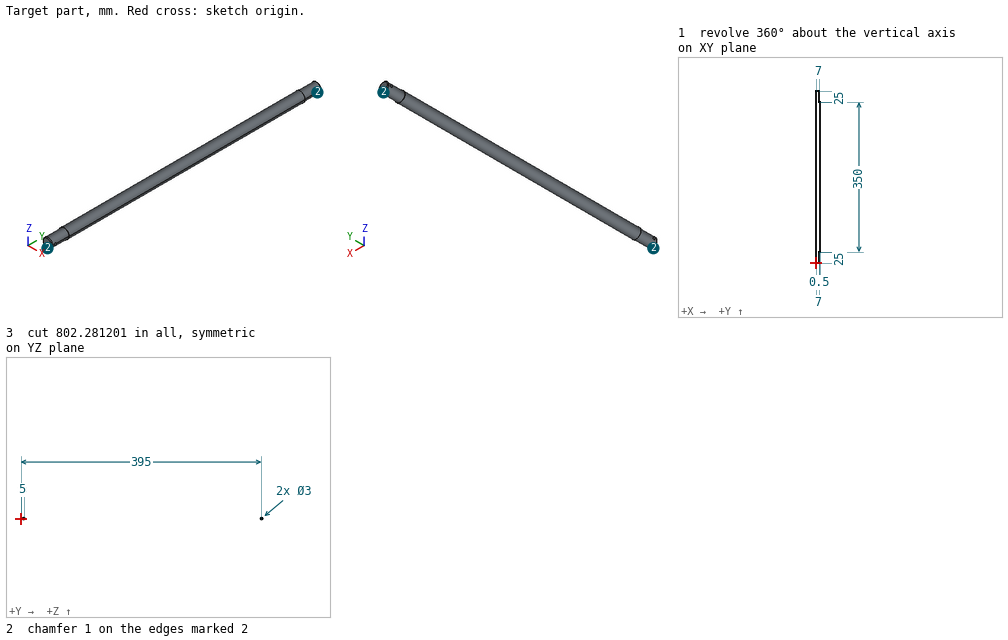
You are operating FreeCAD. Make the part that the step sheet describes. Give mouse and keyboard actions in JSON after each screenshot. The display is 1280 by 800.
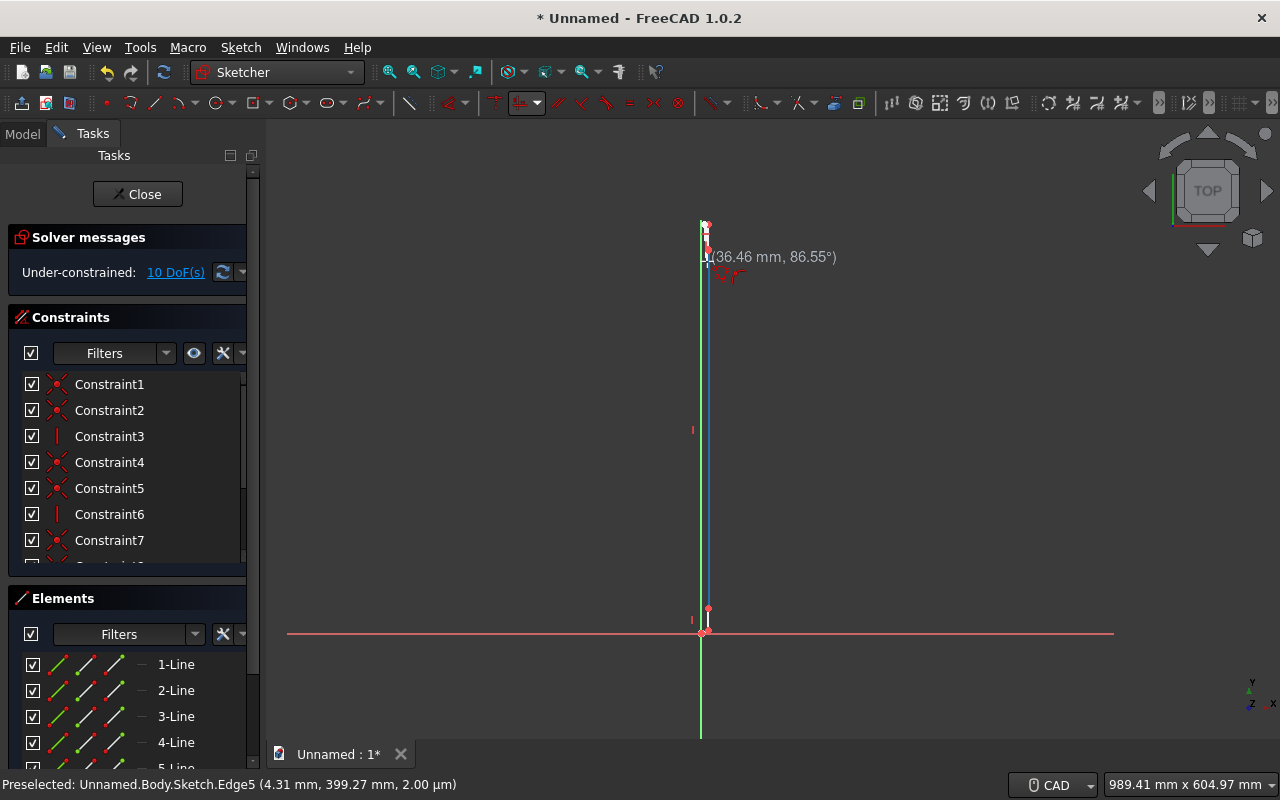
{"action": "scroll", "coordinate": [701, 634], "scroll_direction": "up", "scroll_amount": 8}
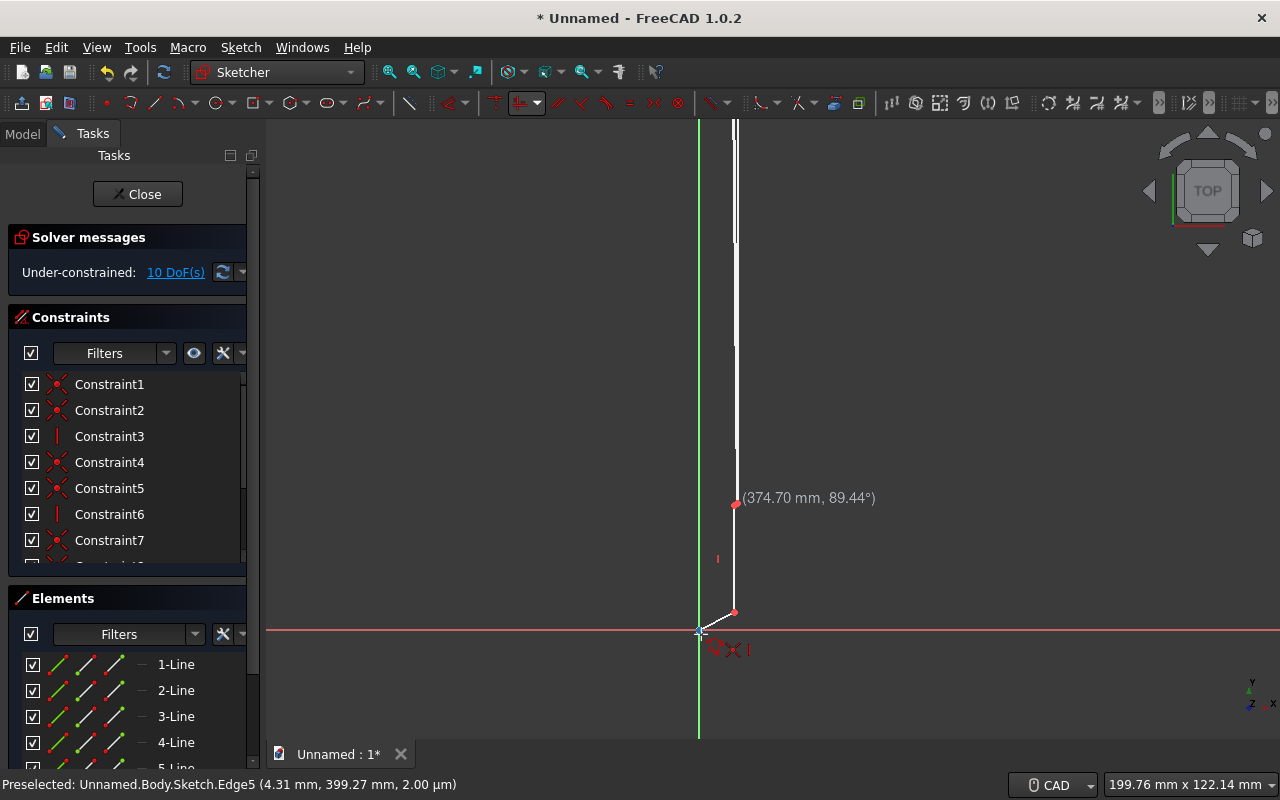
{"action": "left_click", "coordinate": [699, 630]}
{"action": "key", "text": "Escape"}
{"action": "key", "text": "Escape"}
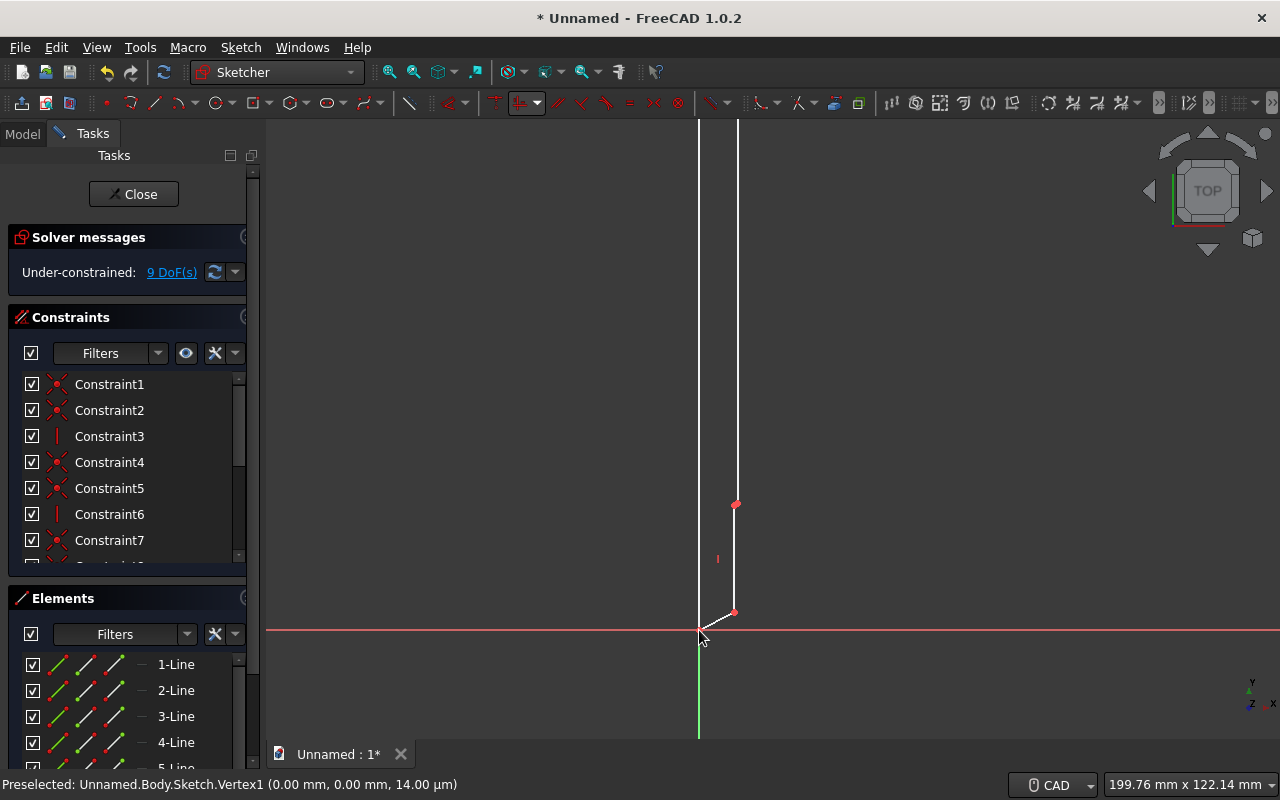
{"action": "left_click", "coordinate": [724, 618]}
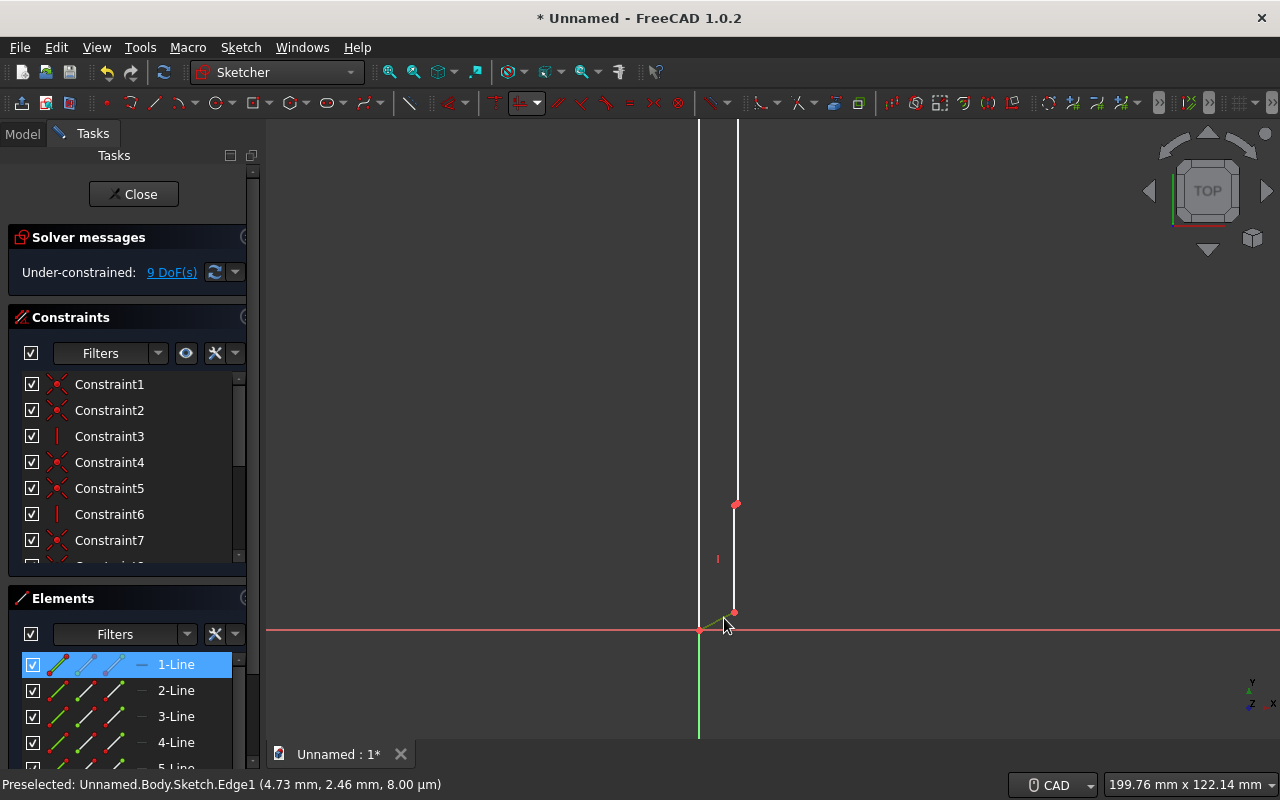
{"action": "left_click", "coordinate": [540, 104]}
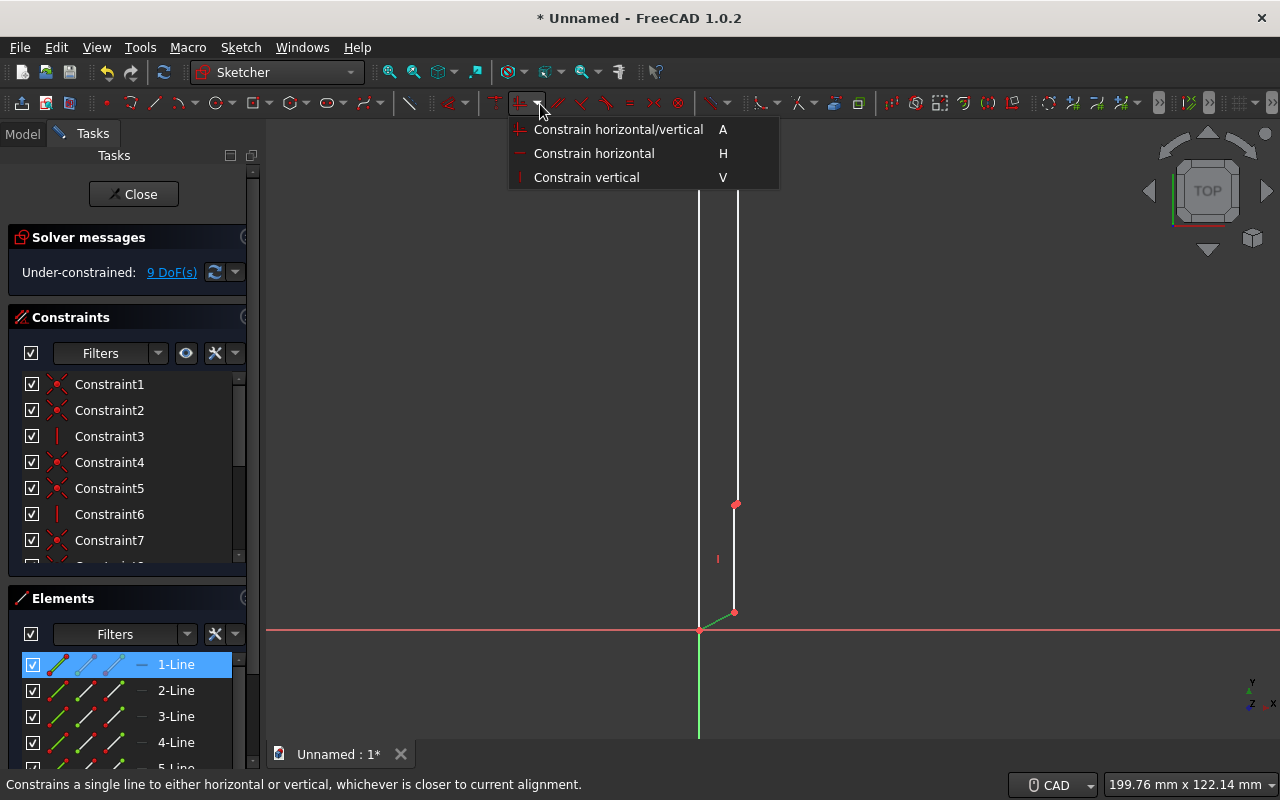
{"action": "left_click", "coordinate": [644, 153]}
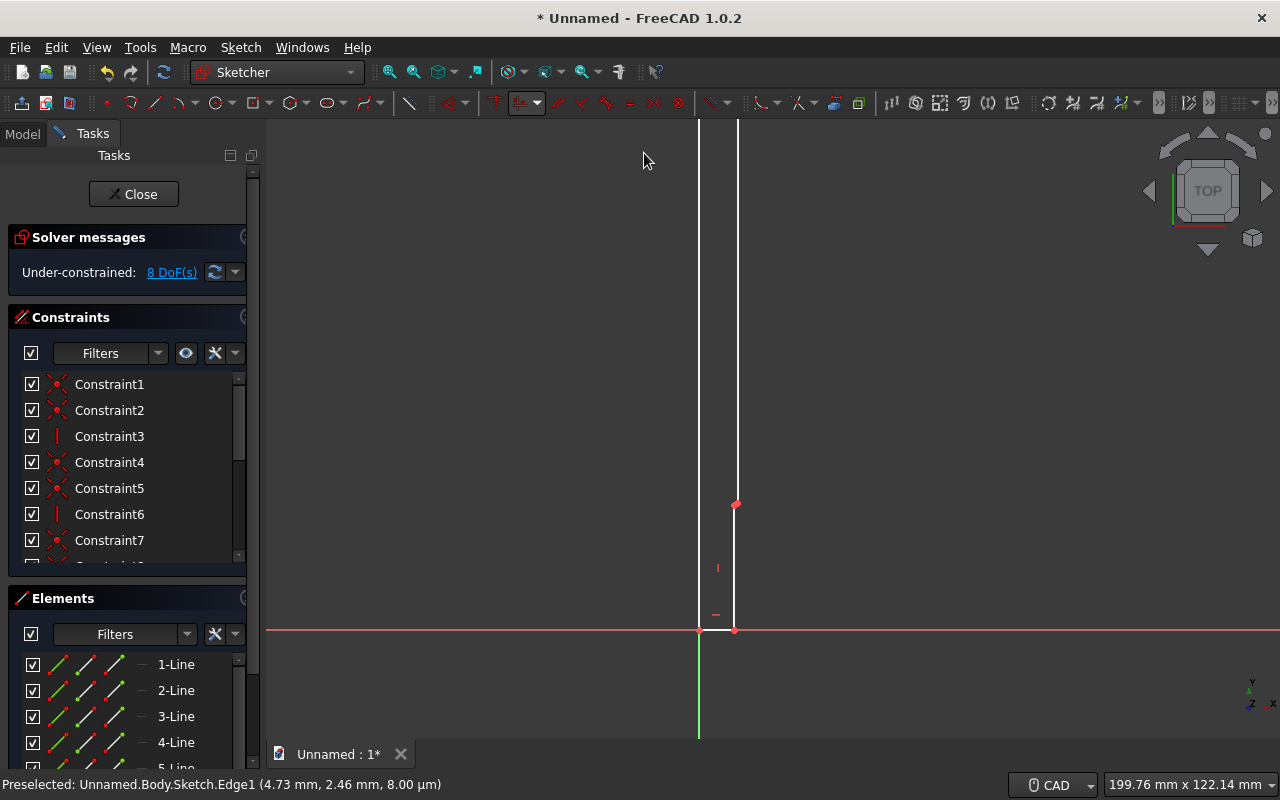
{"action": "scroll", "coordinate": [736, 504], "scroll_direction": "up", "scroll_amount": 6}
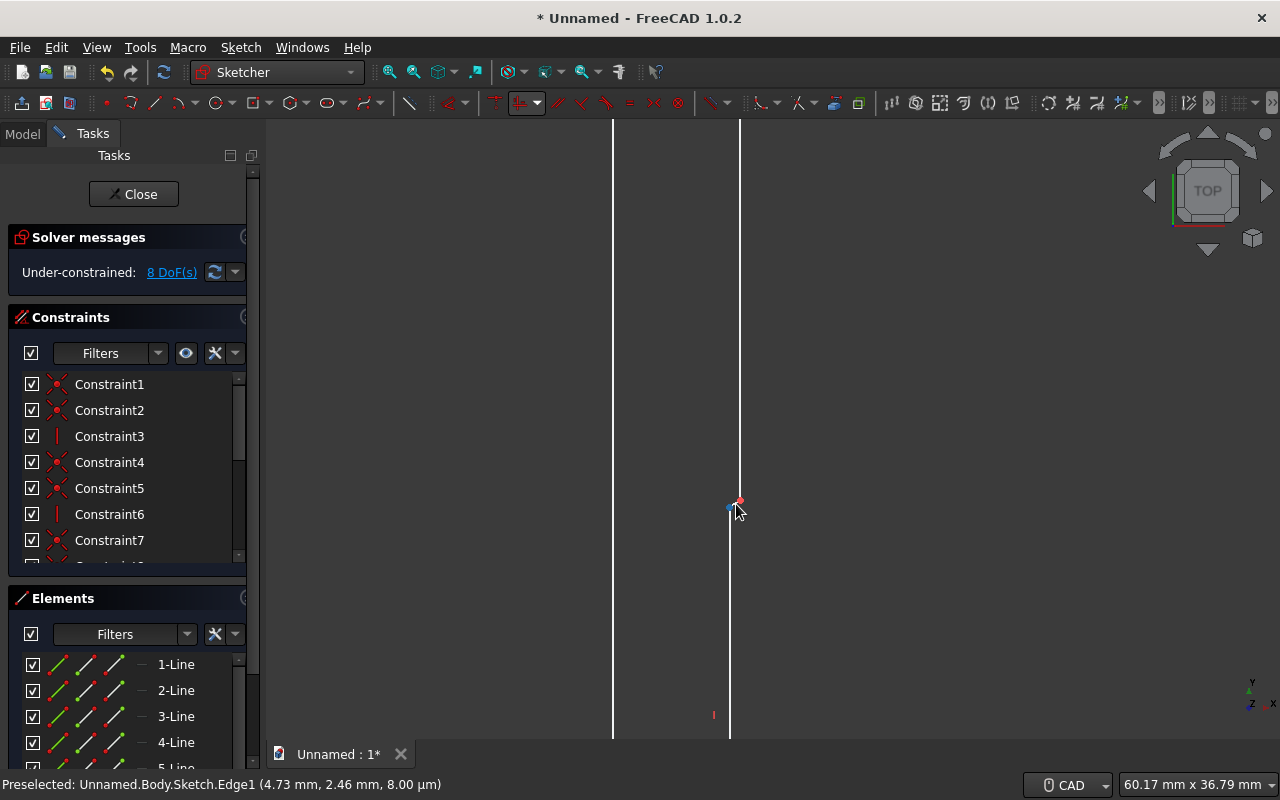
{"action": "left_click", "coordinate": [735, 504]}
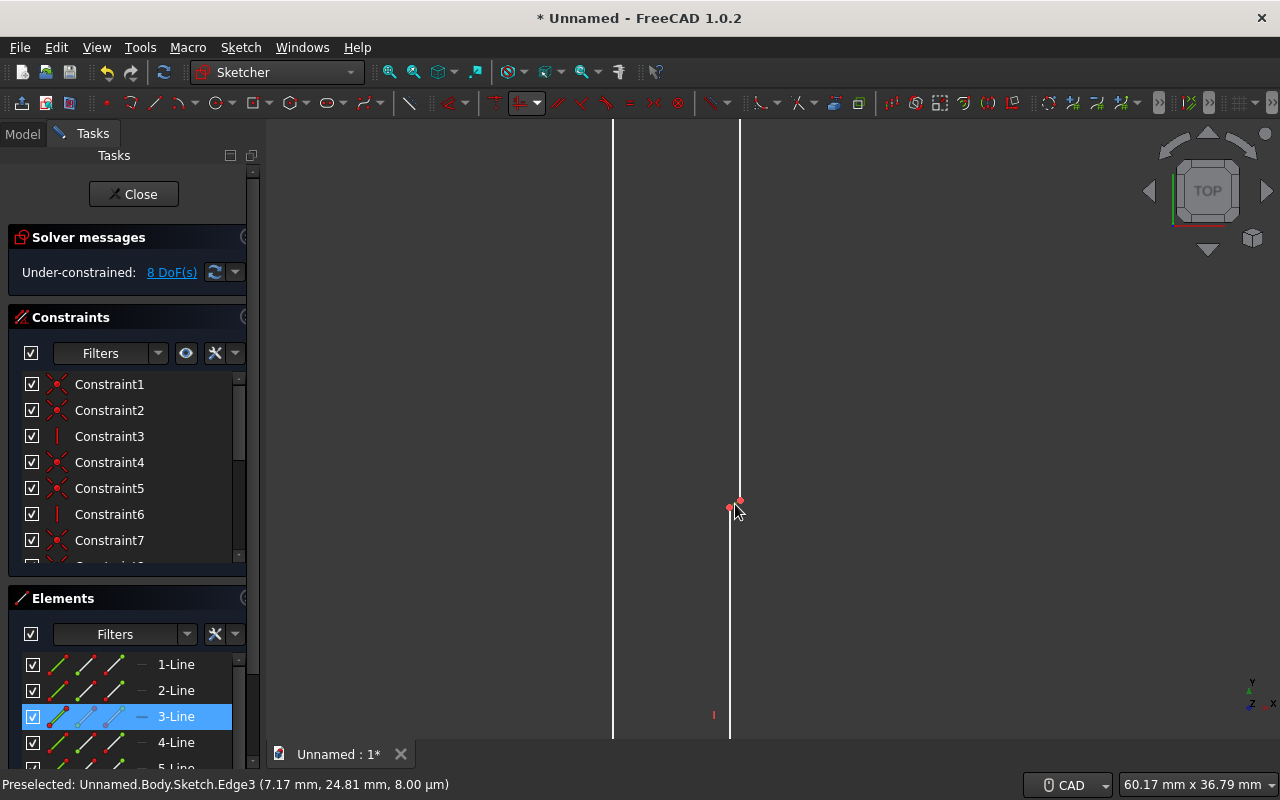
{"action": "left_click", "coordinate": [540, 104]}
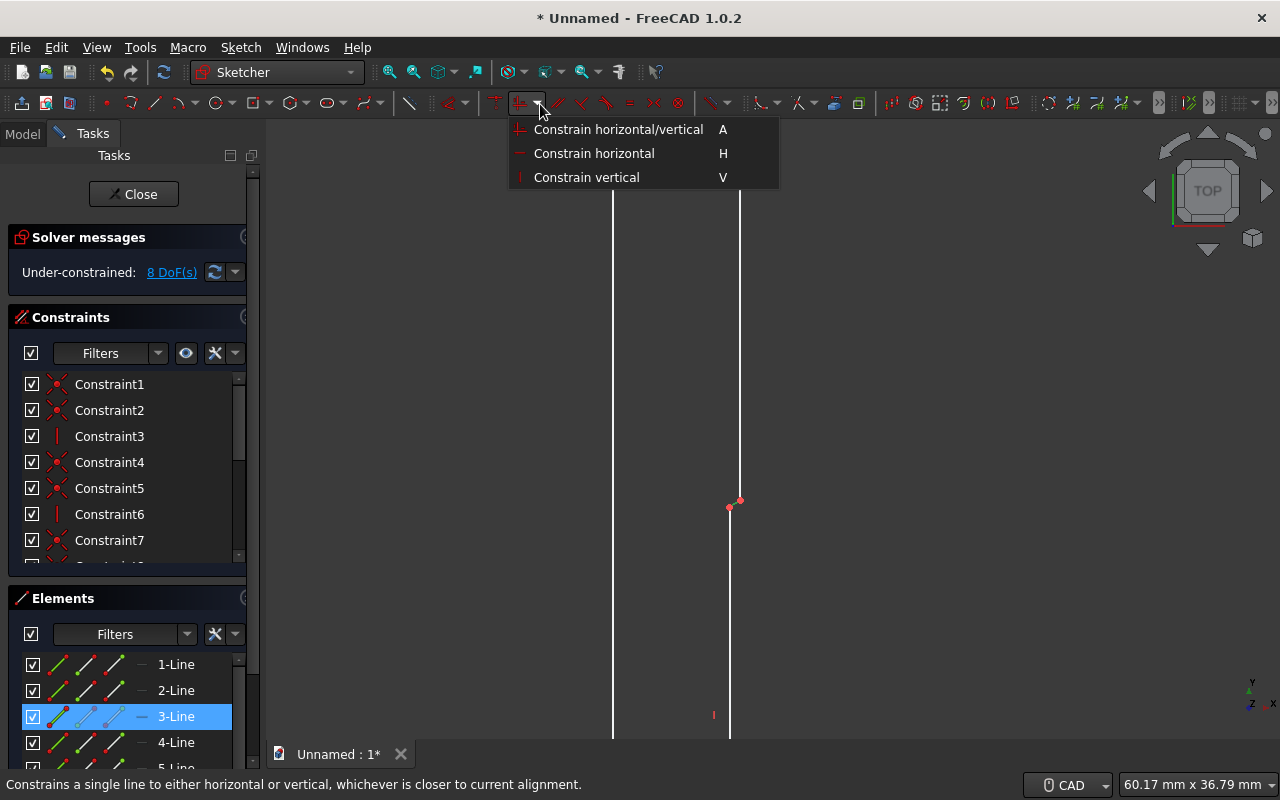
{"action": "left_click", "coordinate": [644, 153]}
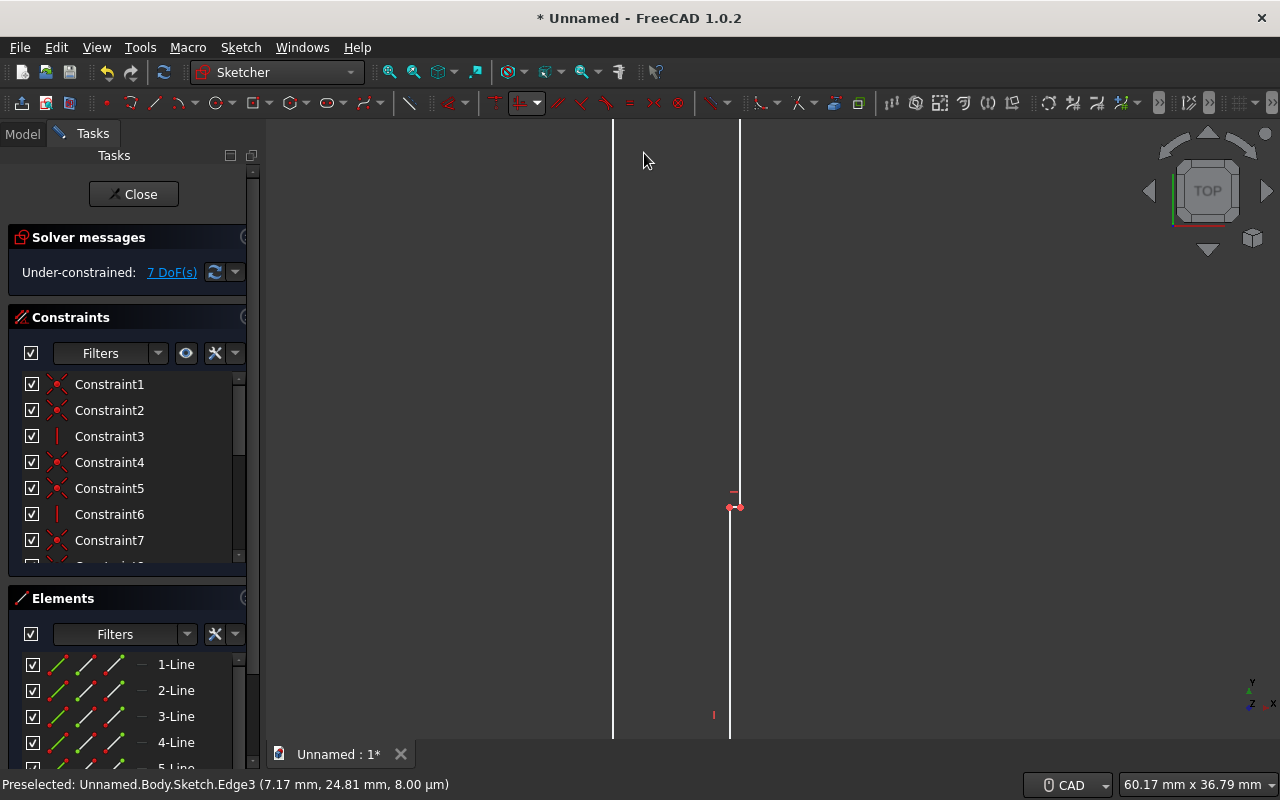
{"action": "scroll", "coordinate": [706, 615], "scroll_direction": "down", "scroll_amount": 14}